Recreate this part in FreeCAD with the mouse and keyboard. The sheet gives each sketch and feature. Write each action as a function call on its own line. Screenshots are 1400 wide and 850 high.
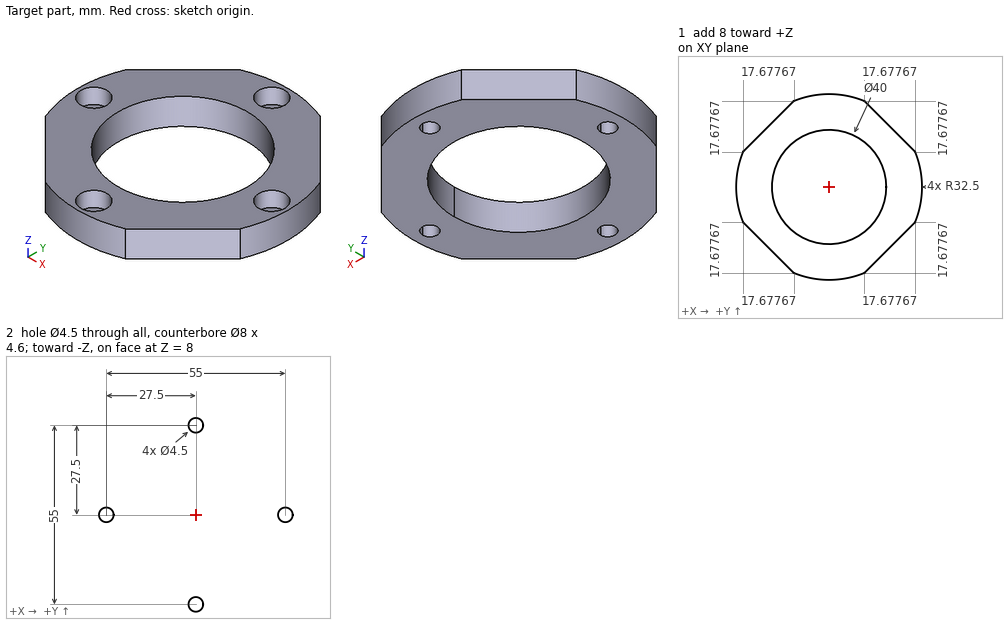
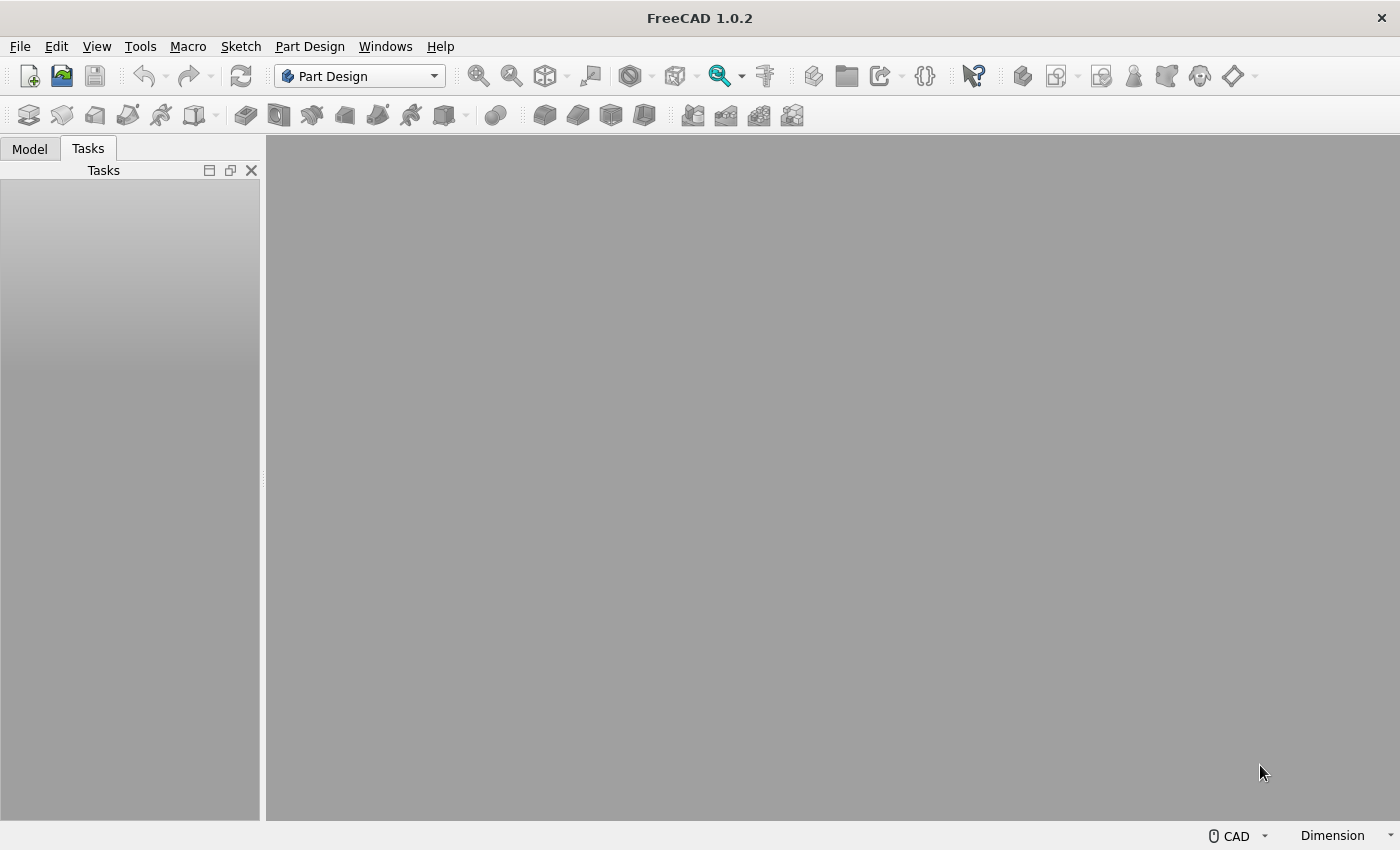
click(29, 76)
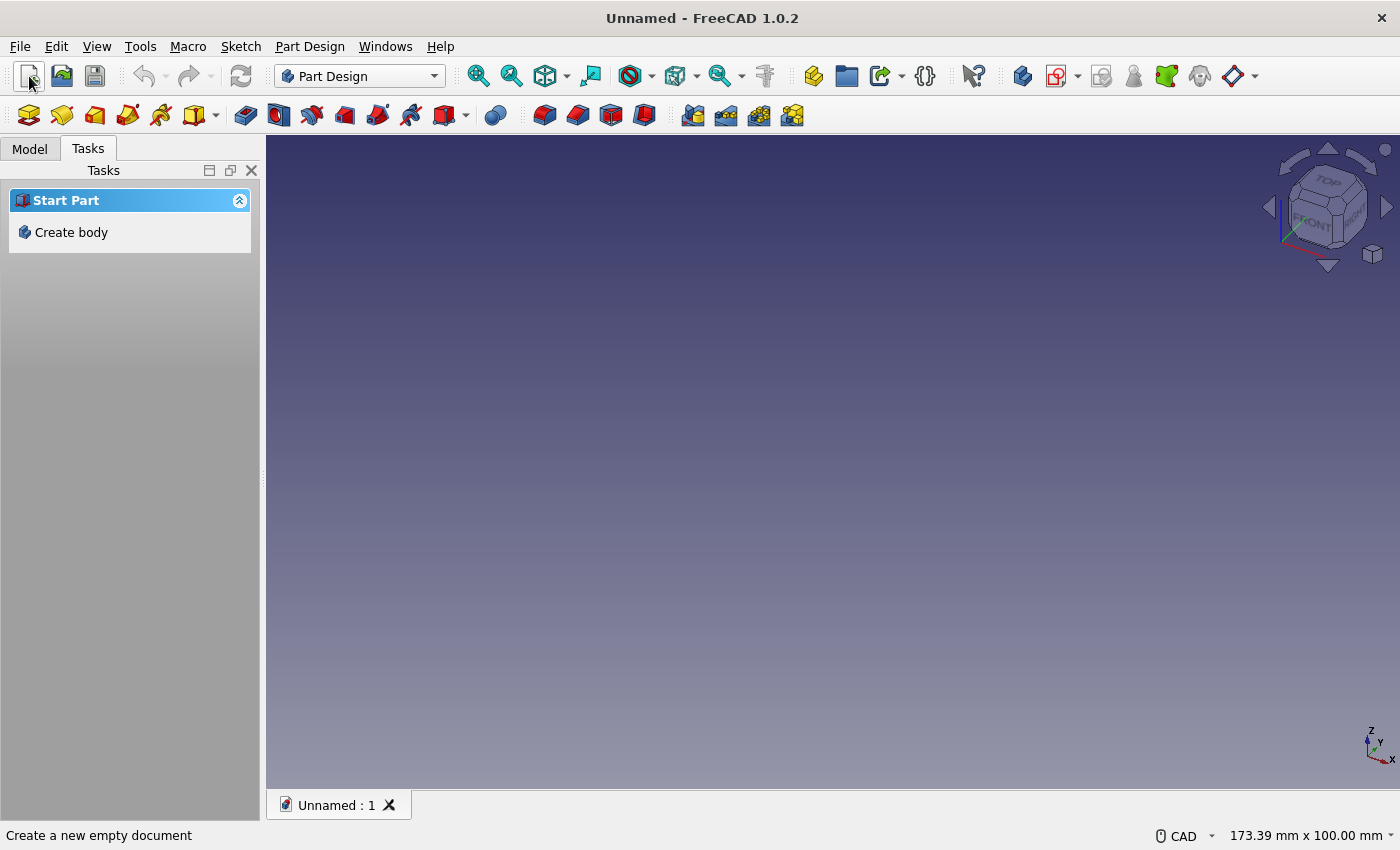
click(1056, 76)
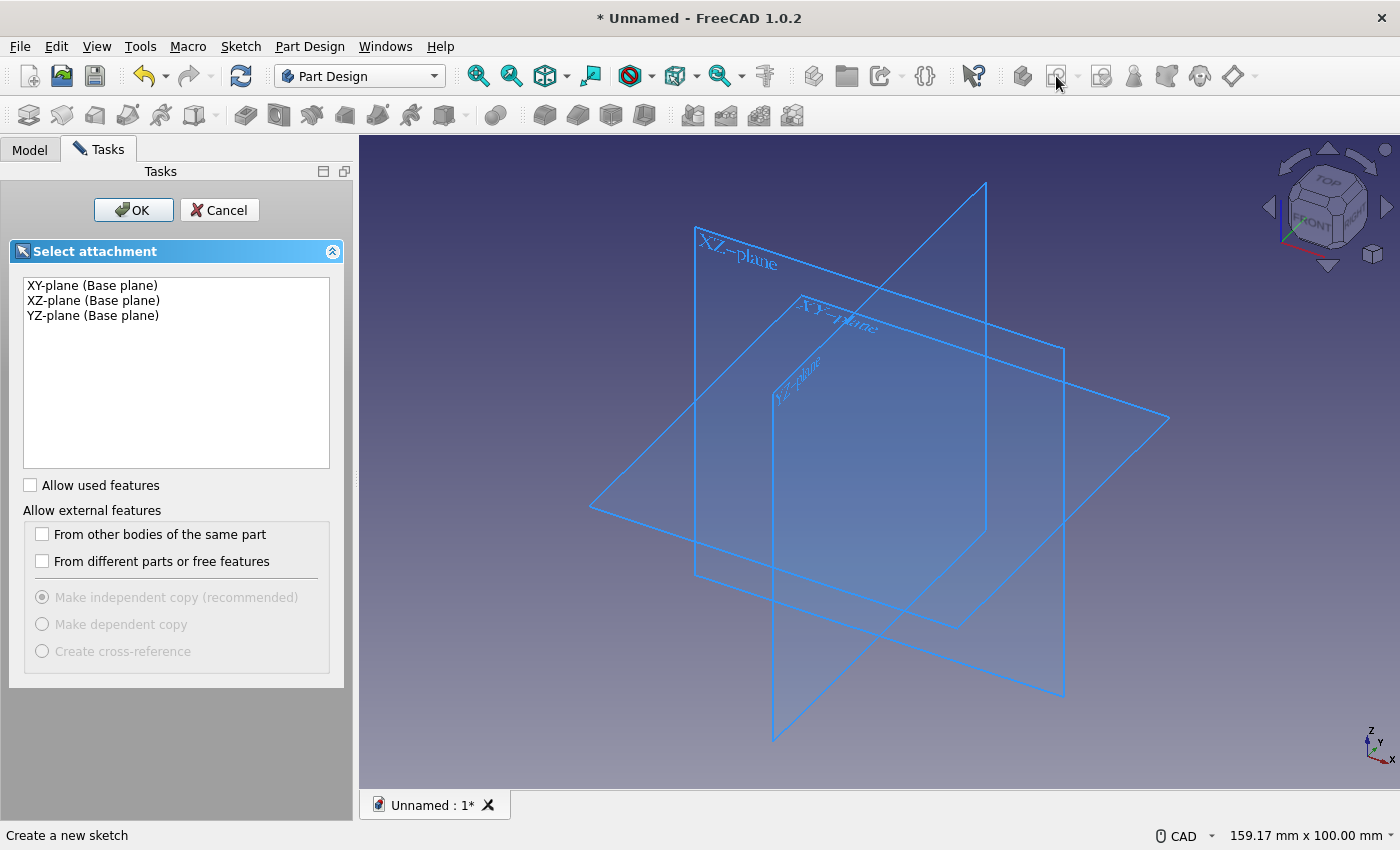
click(84, 286)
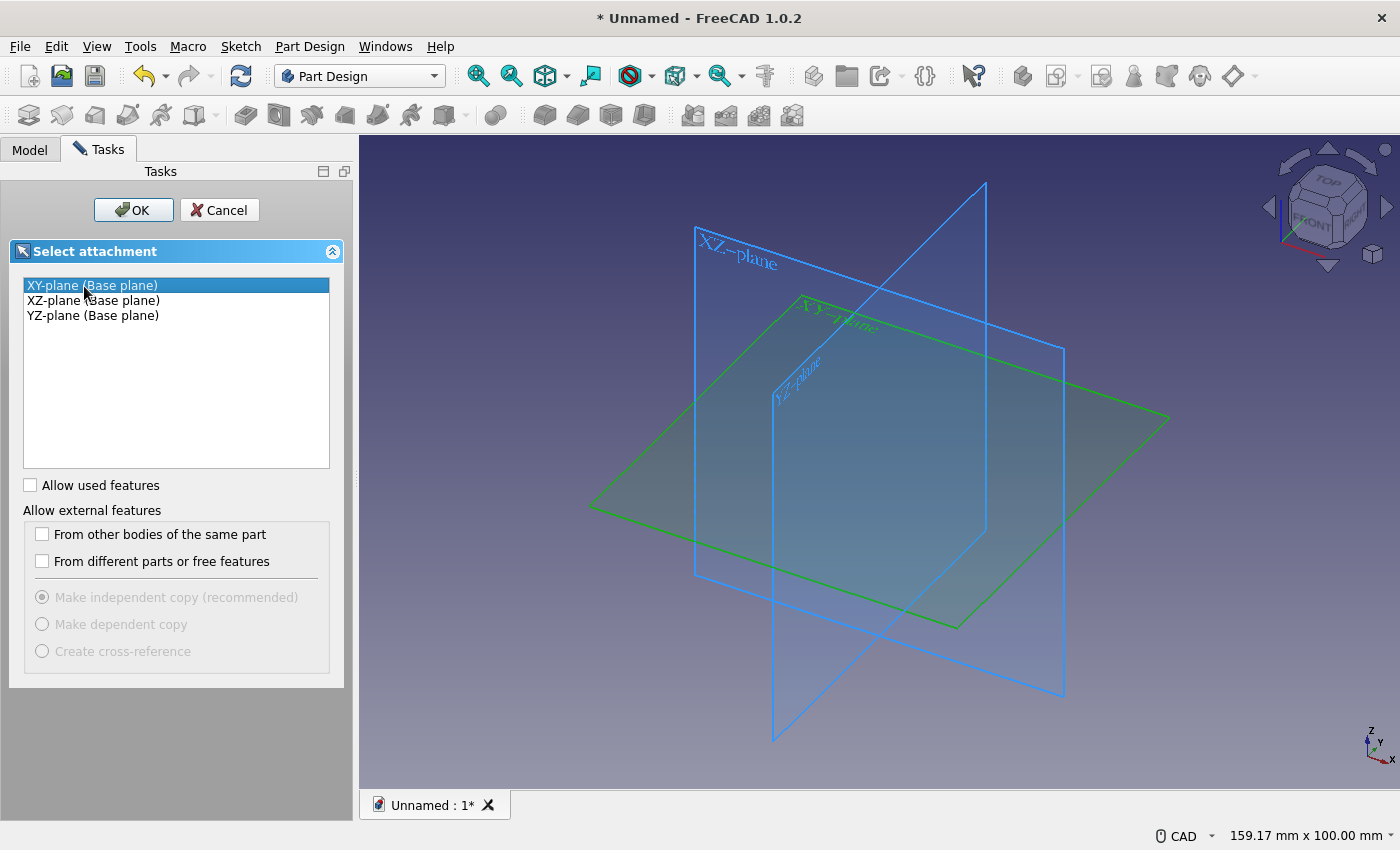
click(134, 210)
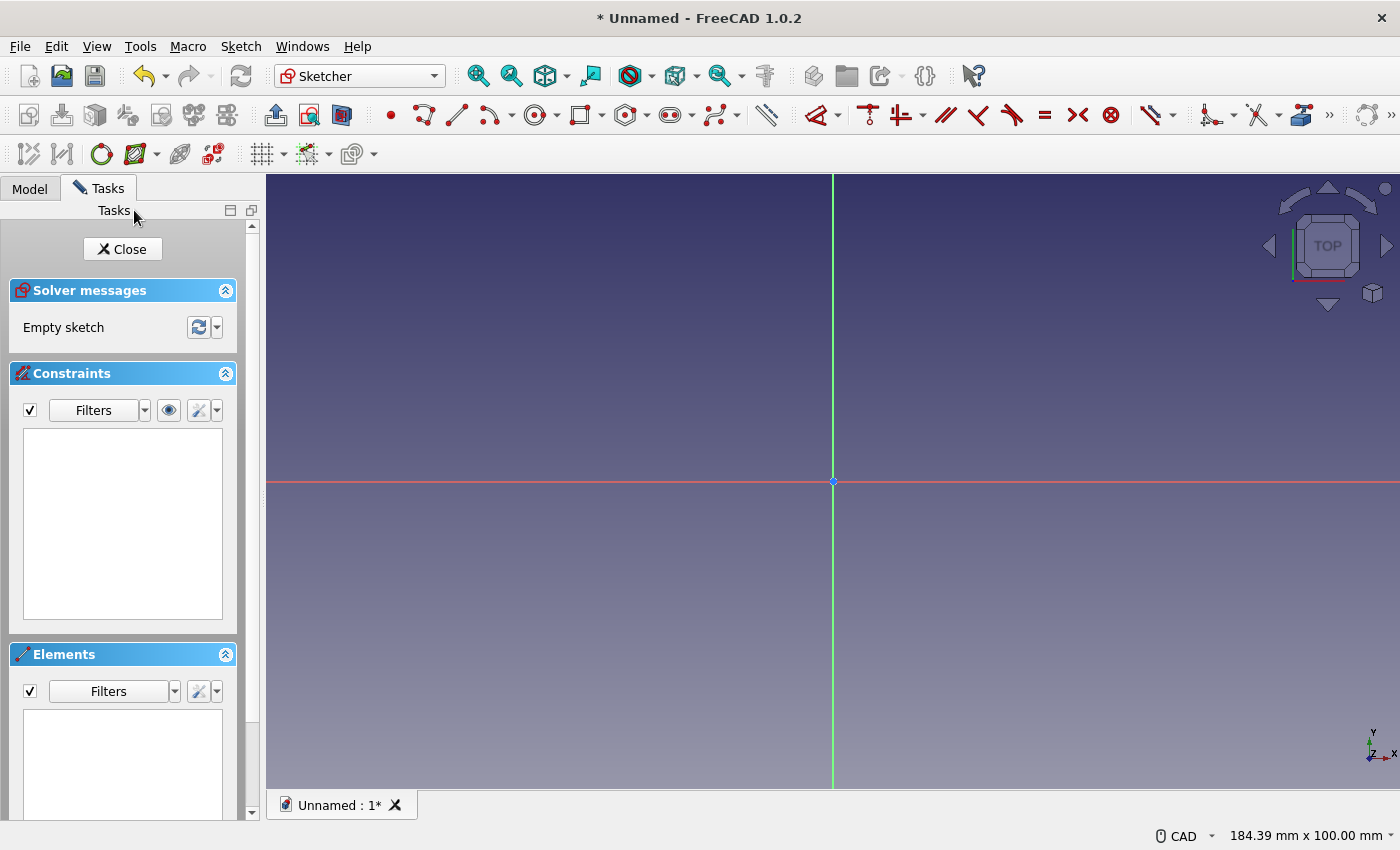
click(457, 116)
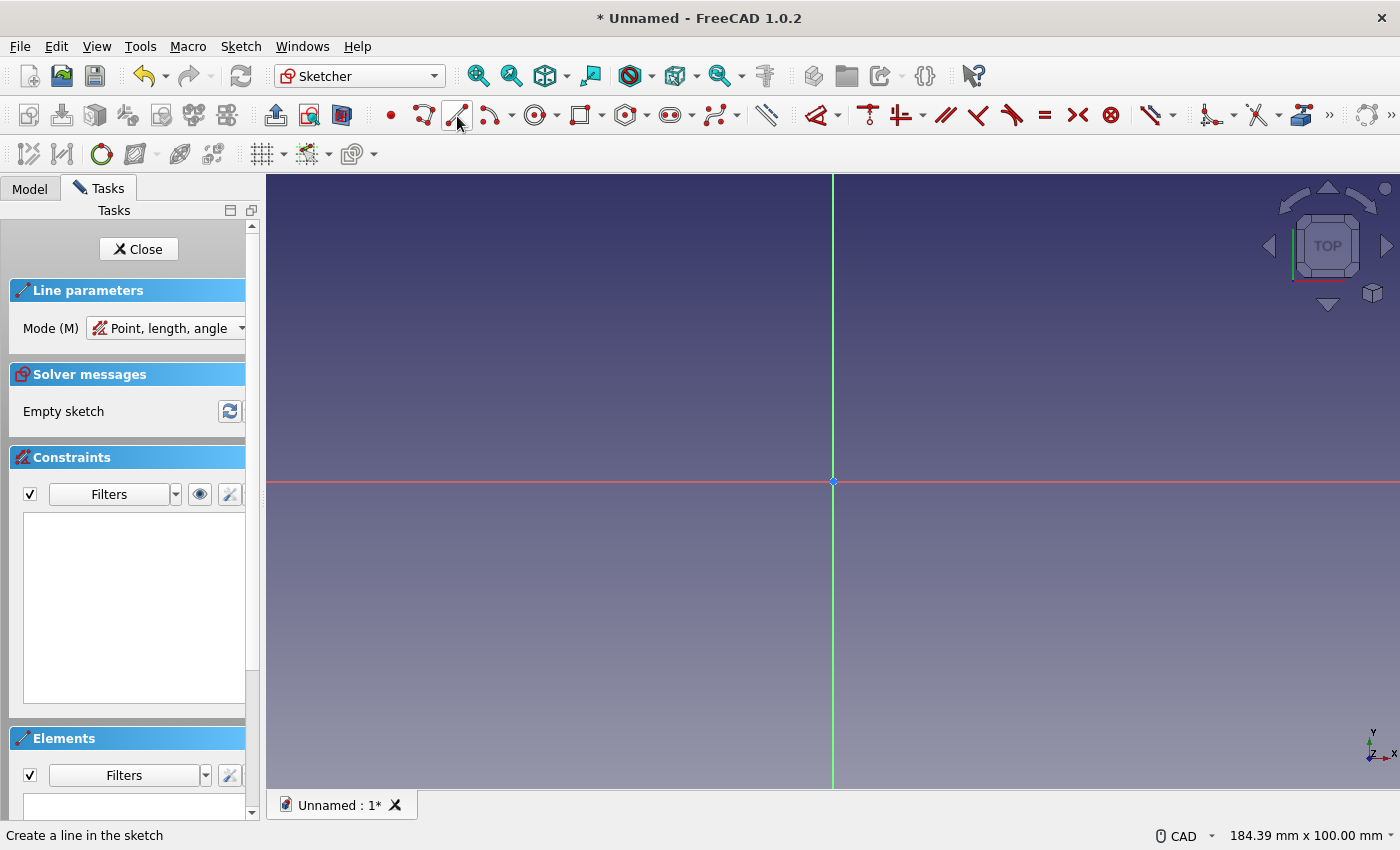
click(648, 558)
click(757, 666)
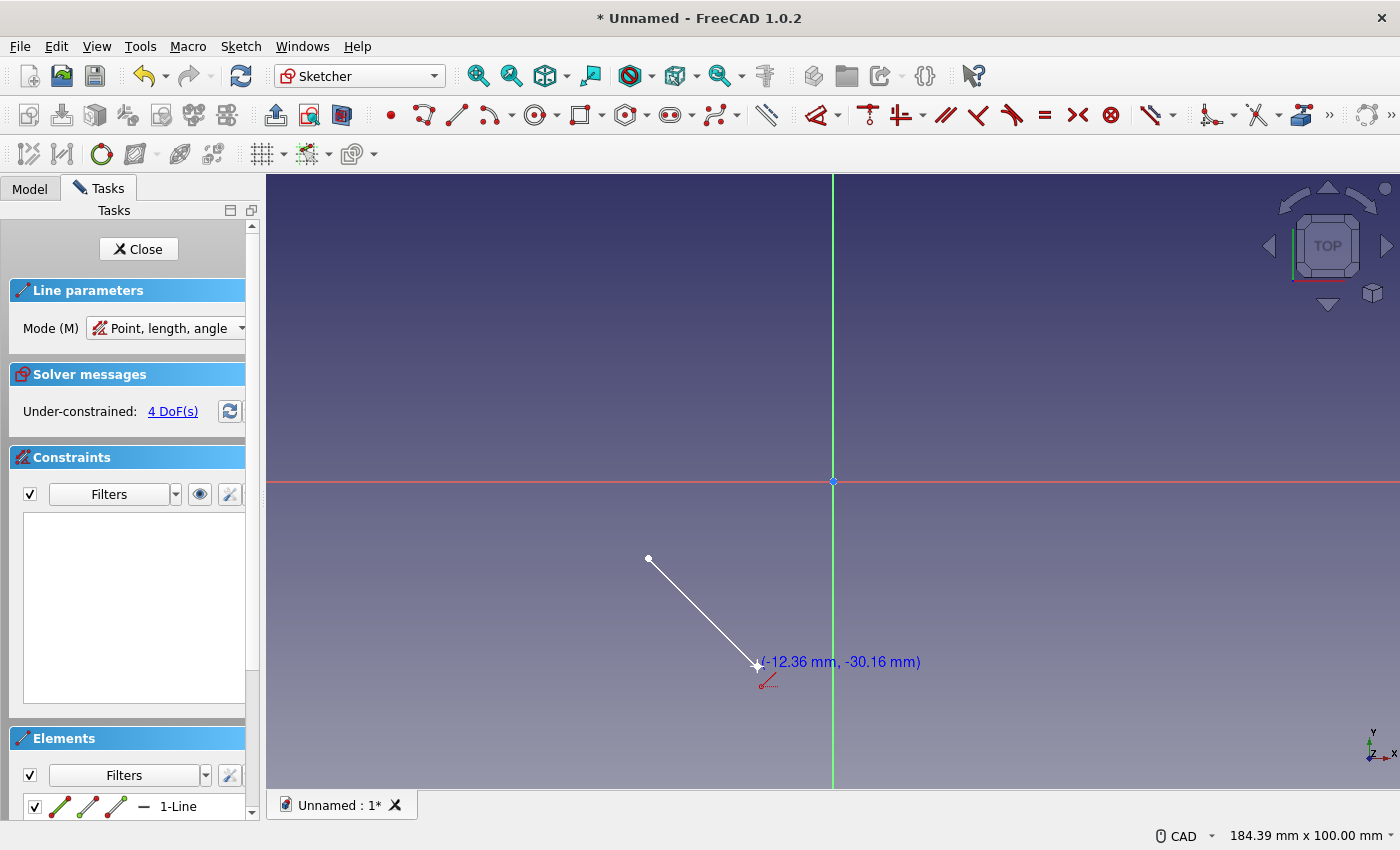
click(909, 666)
click(1018, 558)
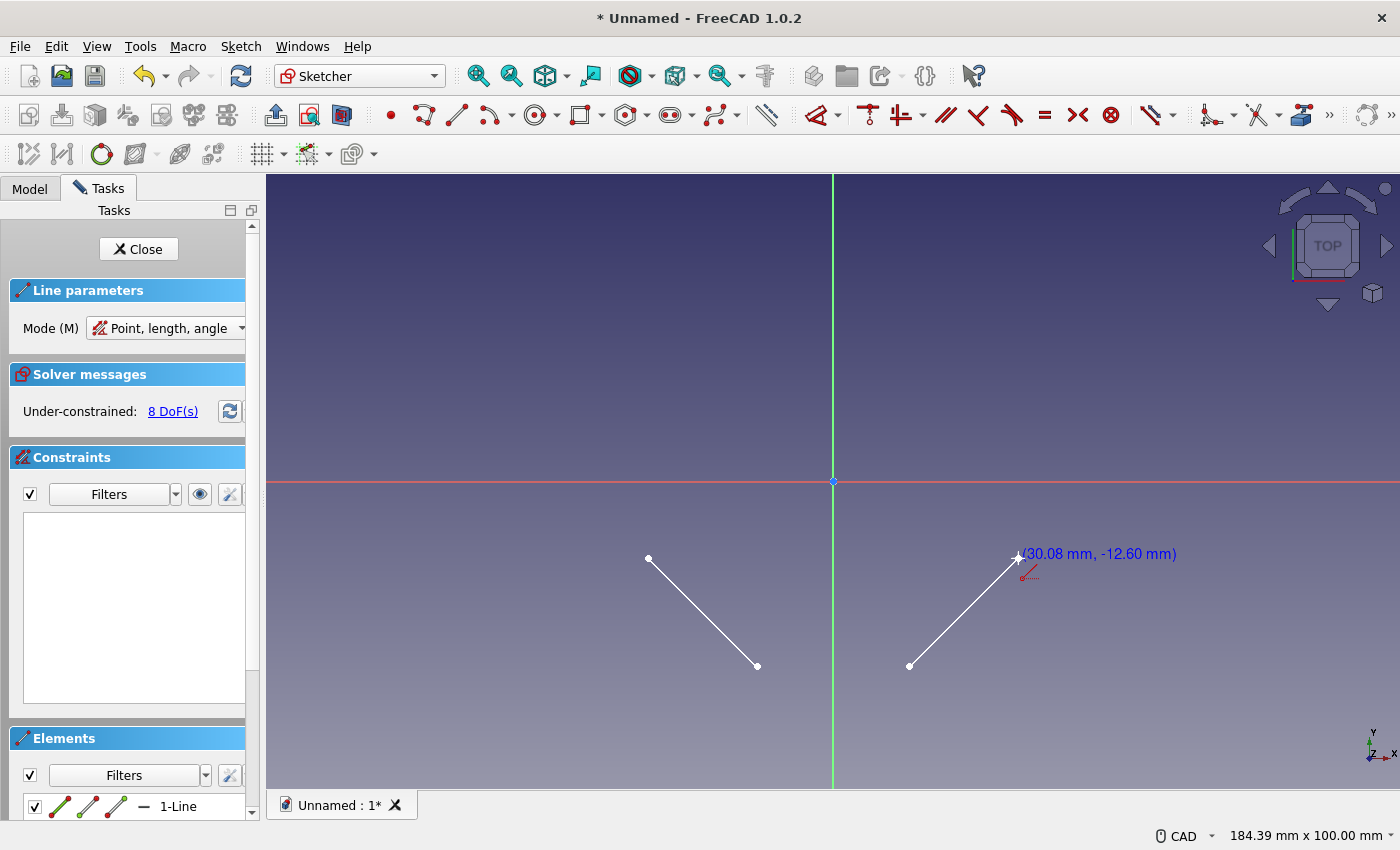
click(1018, 405)
click(909, 297)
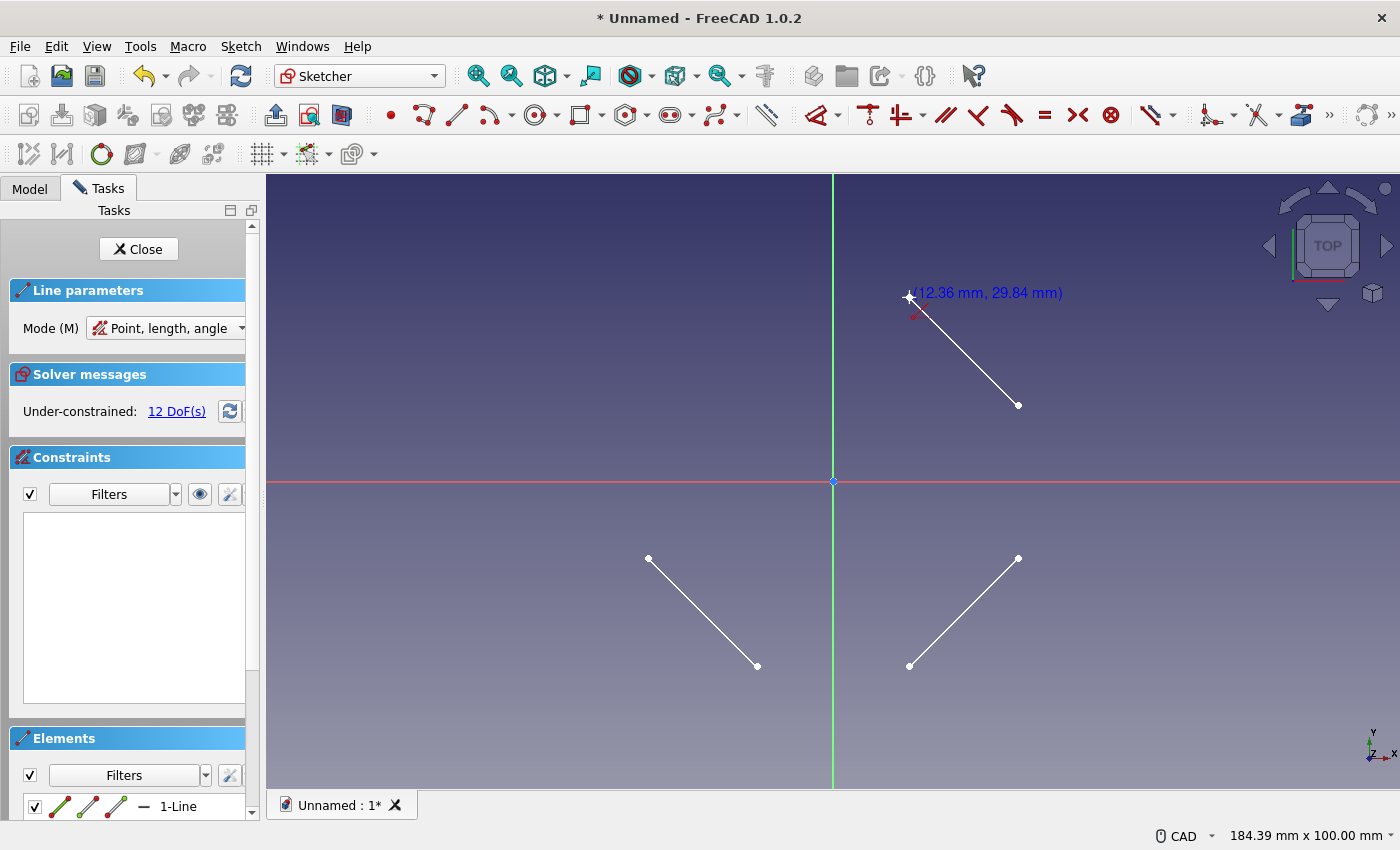
click(757, 297)
click(648, 405)